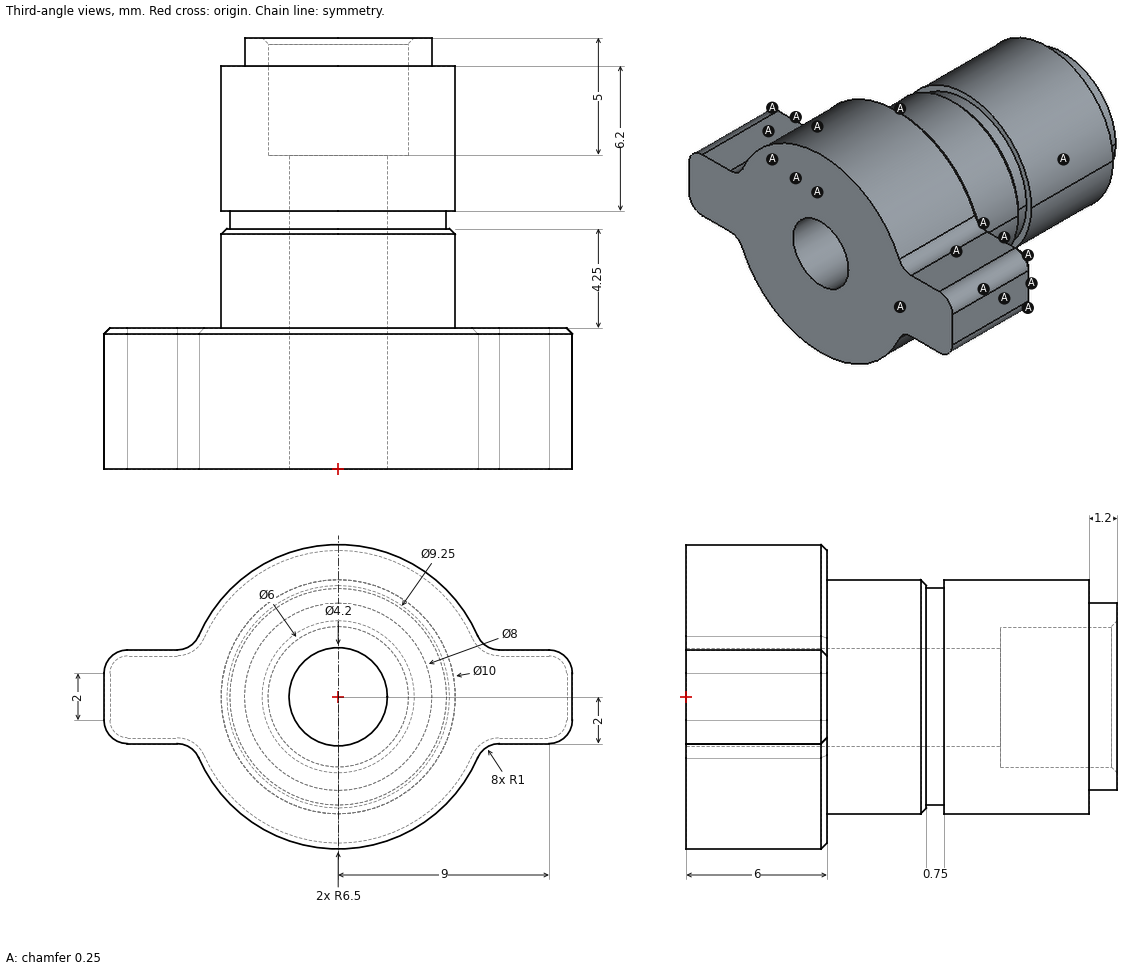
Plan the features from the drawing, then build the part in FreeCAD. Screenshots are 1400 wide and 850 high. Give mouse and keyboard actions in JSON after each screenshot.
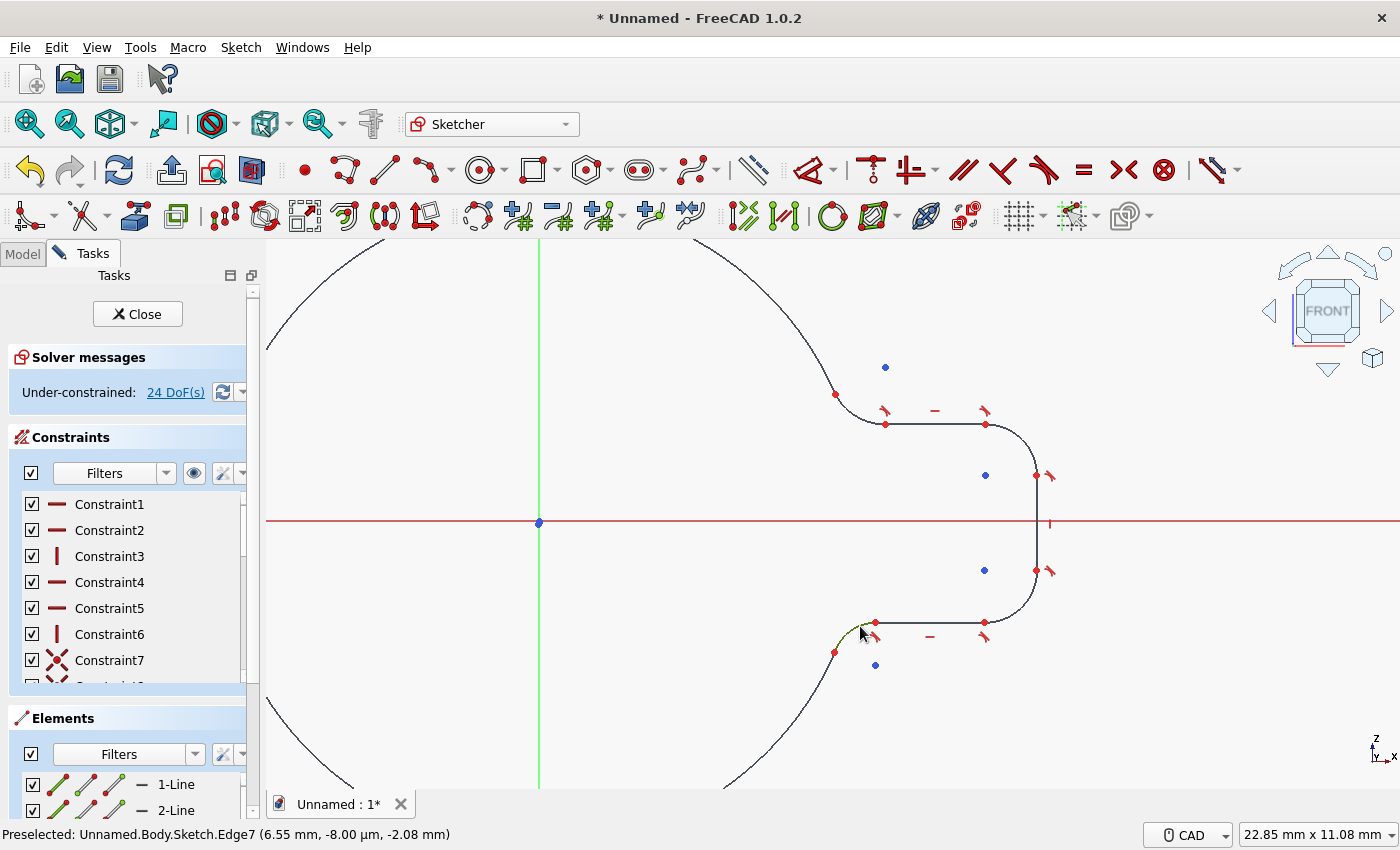
{"action": "scroll", "coordinate": [1039, 505], "scroll_direction": "down", "scroll_amount": 3}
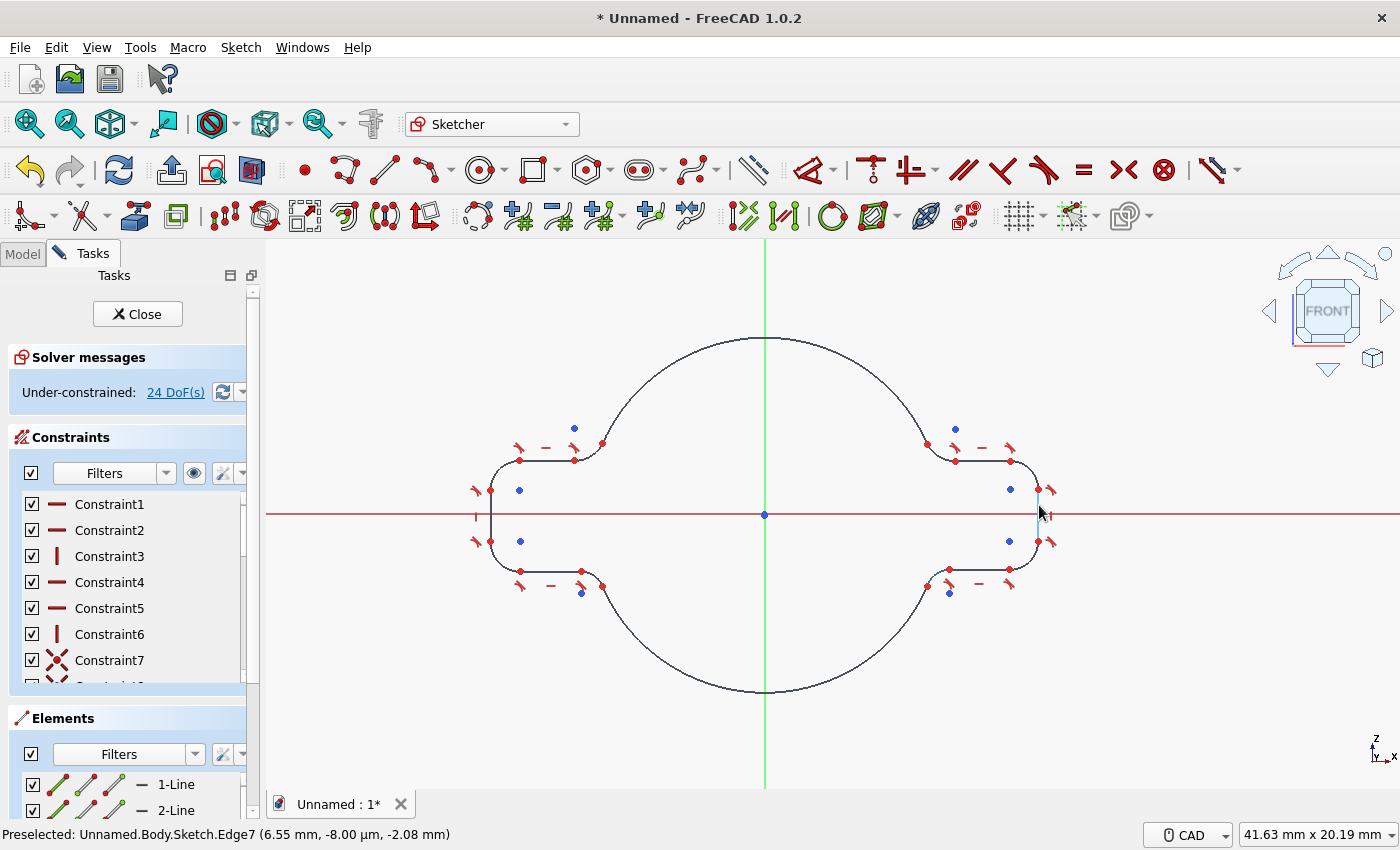
{"action": "left_click", "coordinate": [686, 674]}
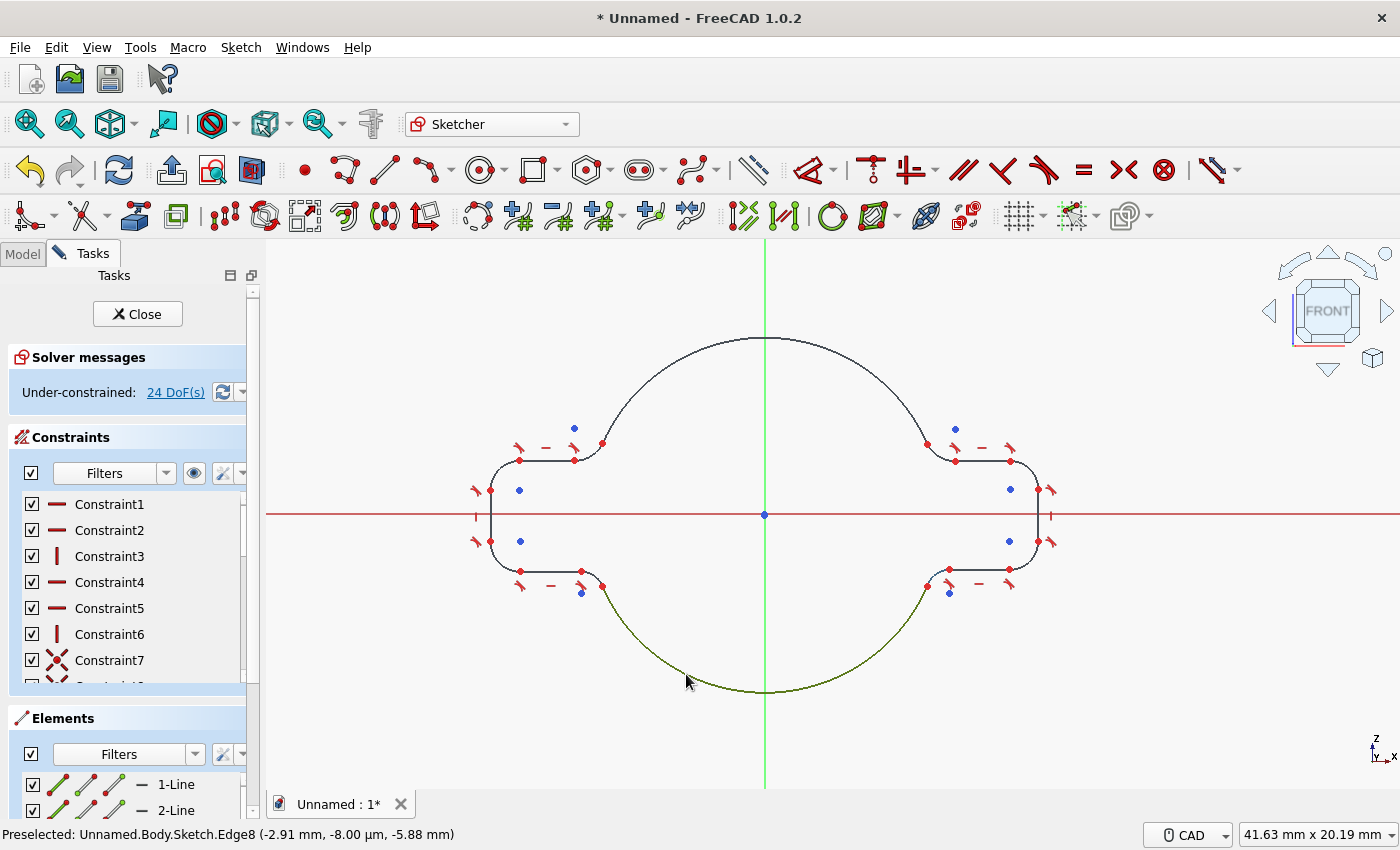
{"action": "left_click", "coordinate": [1044, 170]}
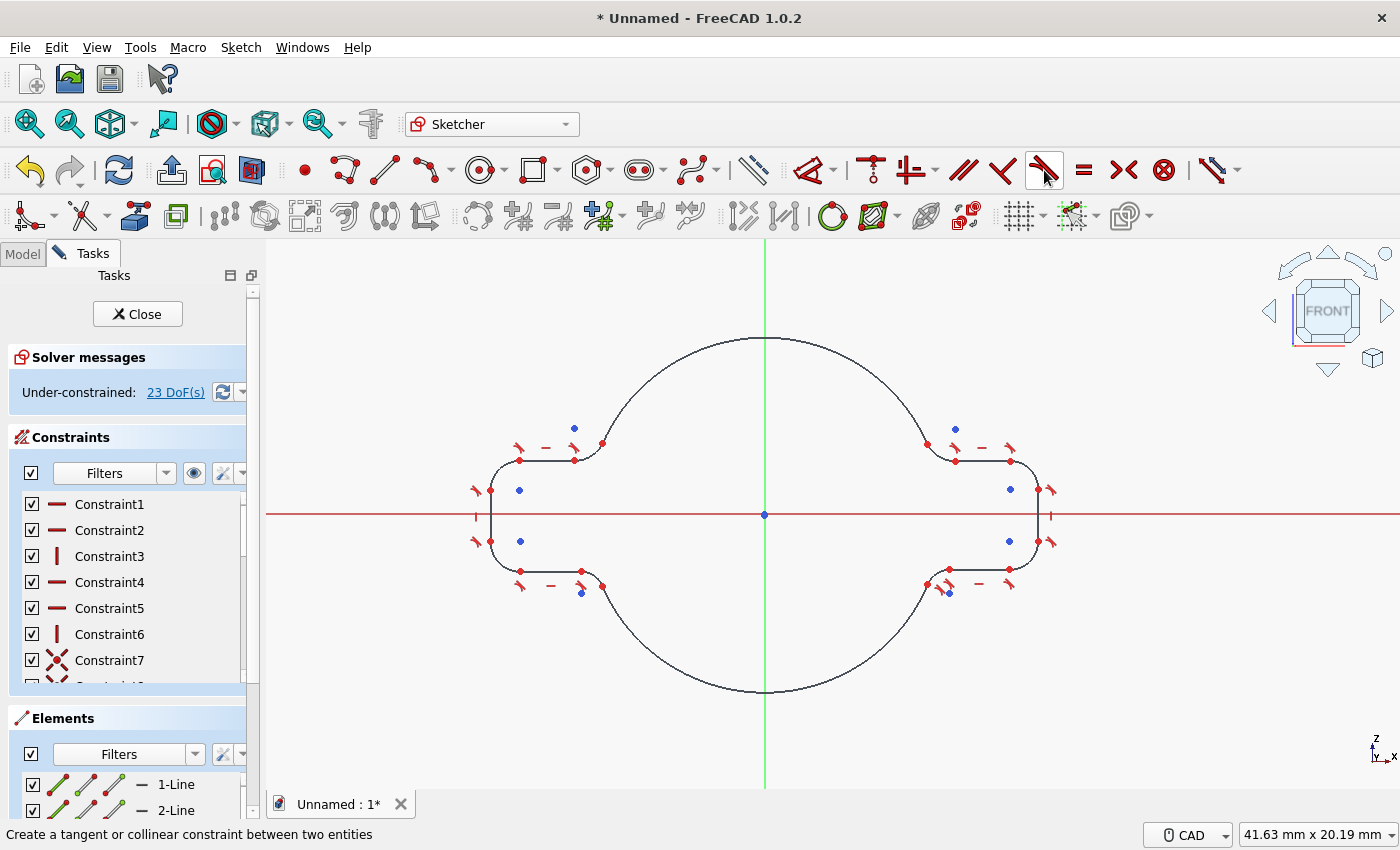
{"action": "left_click", "coordinate": [686, 674]}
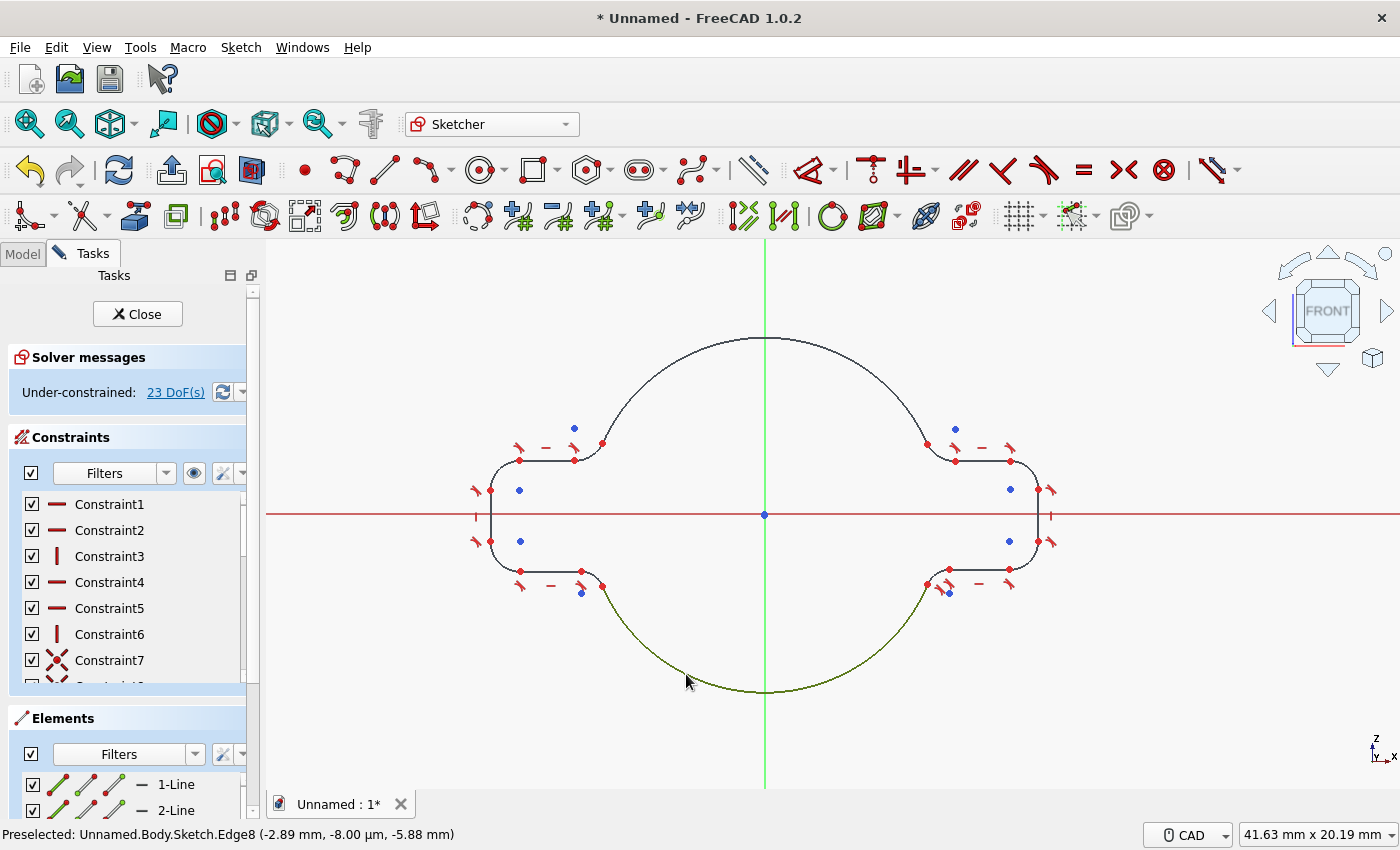
{"action": "left_click", "coordinate": [595, 576]}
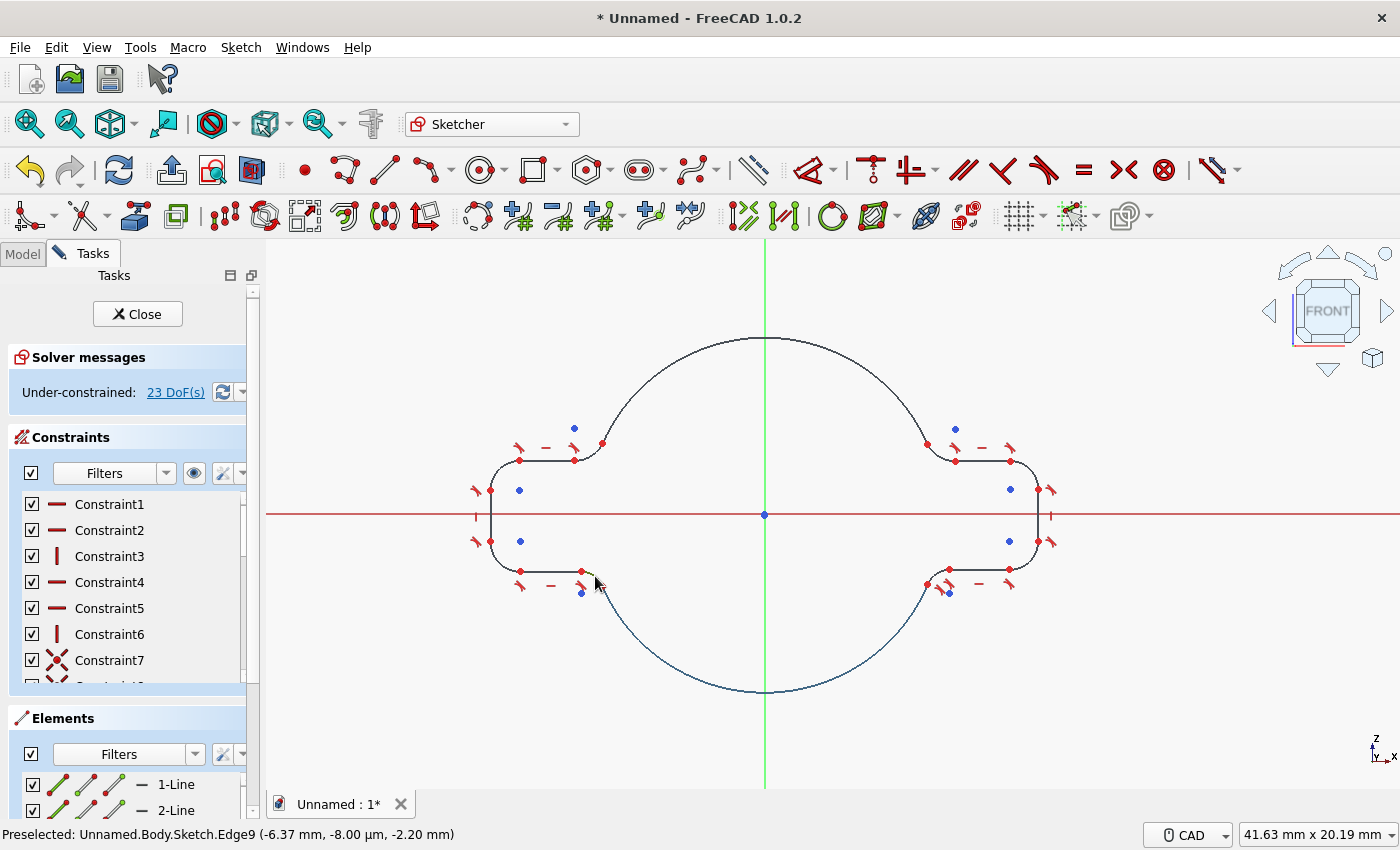
{"action": "left_click", "coordinate": [1044, 170]}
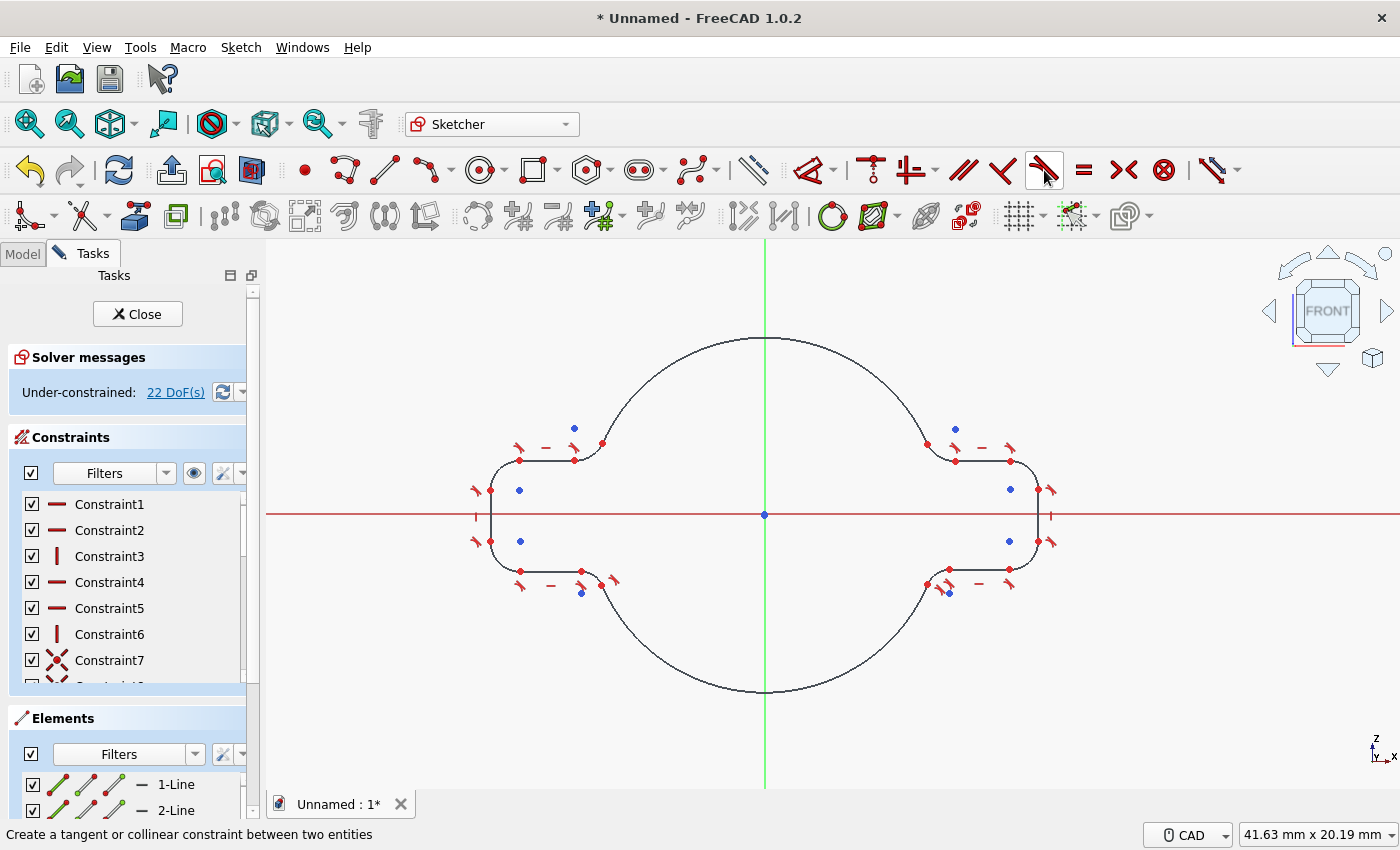
{"action": "scroll", "coordinate": [584, 459], "scroll_direction": "up", "scroll_amount": 2}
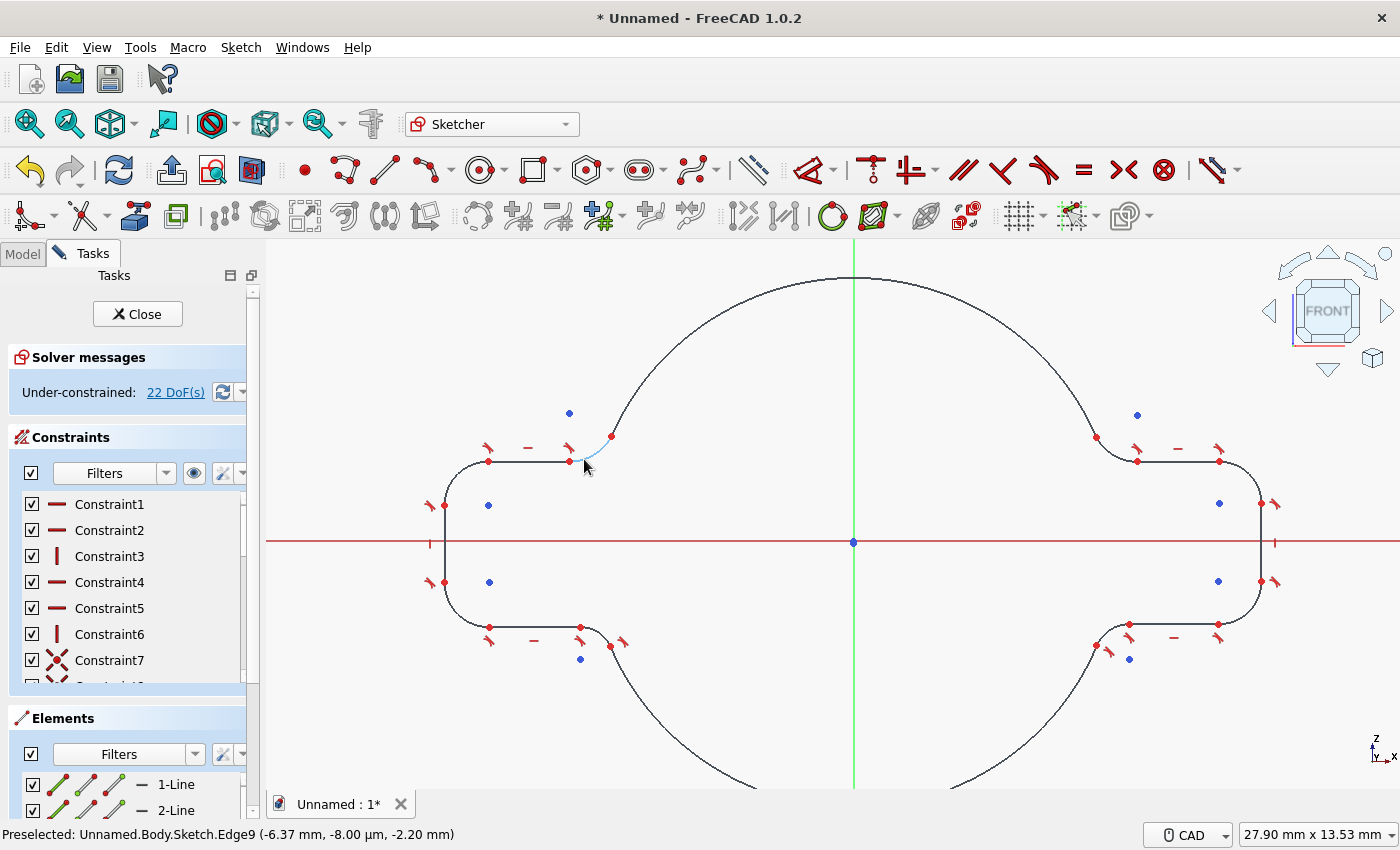
{"action": "left_click", "coordinate": [584, 459]}